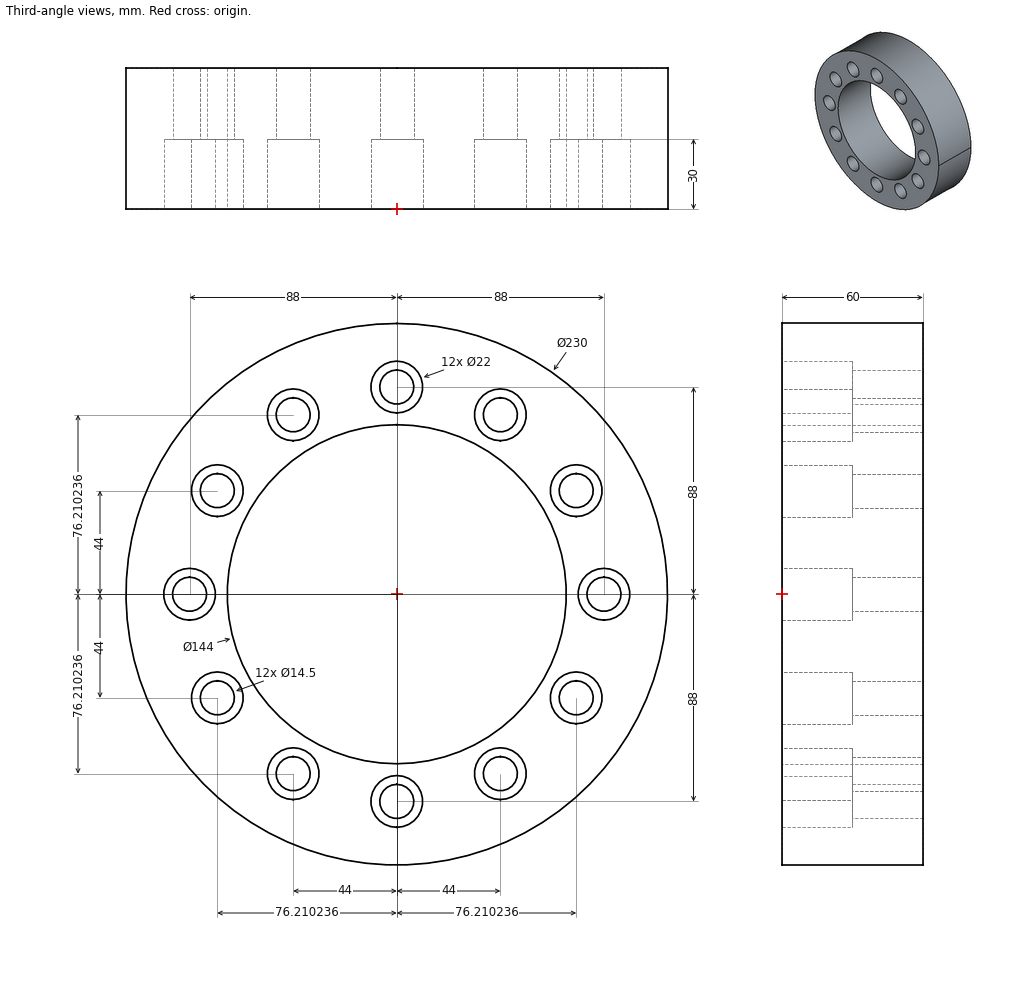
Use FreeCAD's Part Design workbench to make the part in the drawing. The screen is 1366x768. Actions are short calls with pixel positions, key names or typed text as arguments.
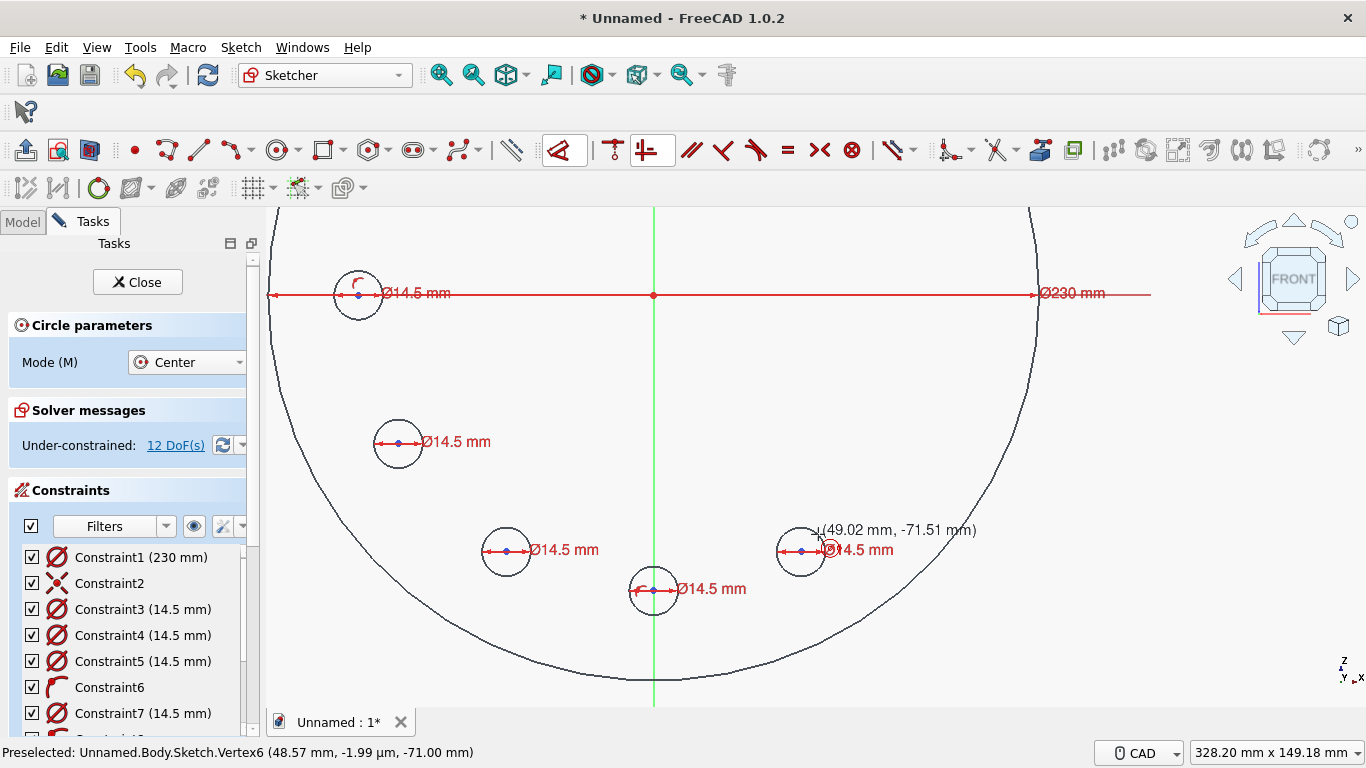
click(909, 443)
move(926, 426)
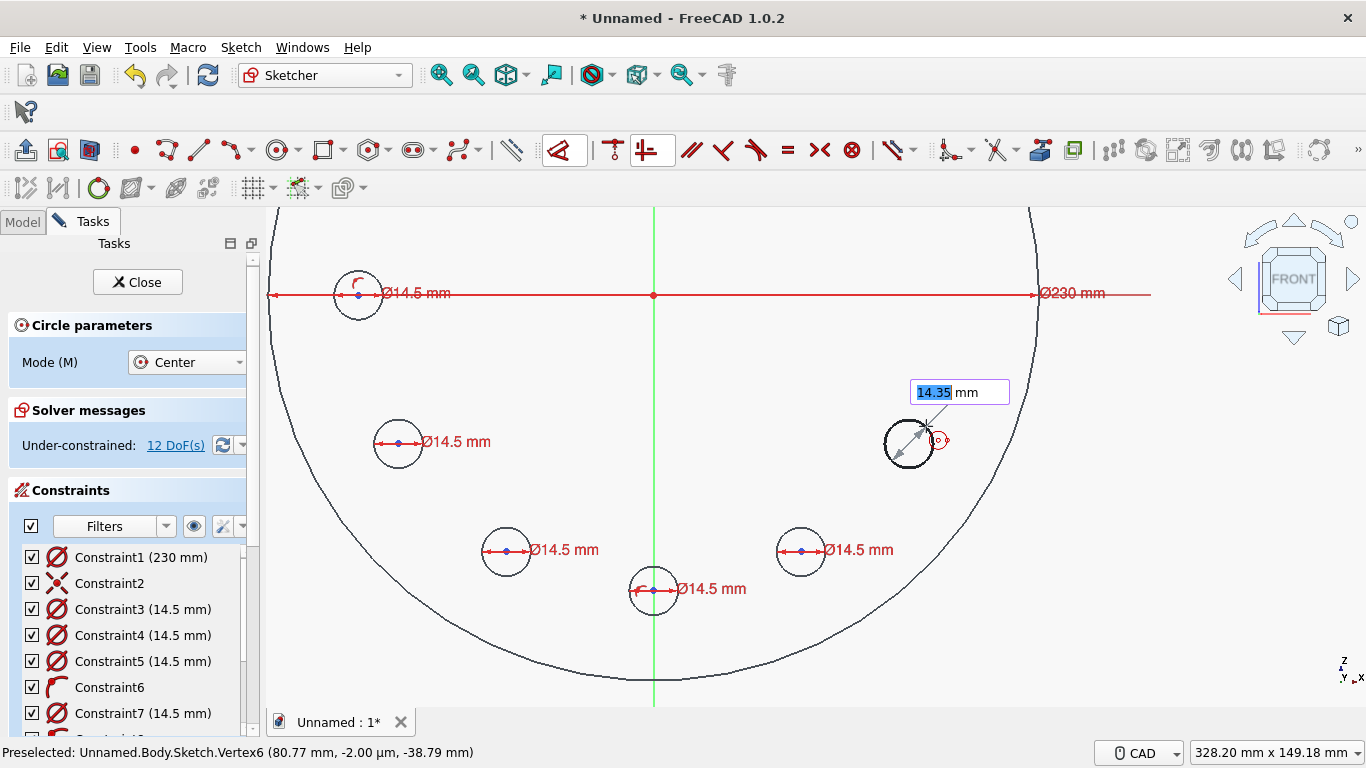
text(14.5)
key(Return)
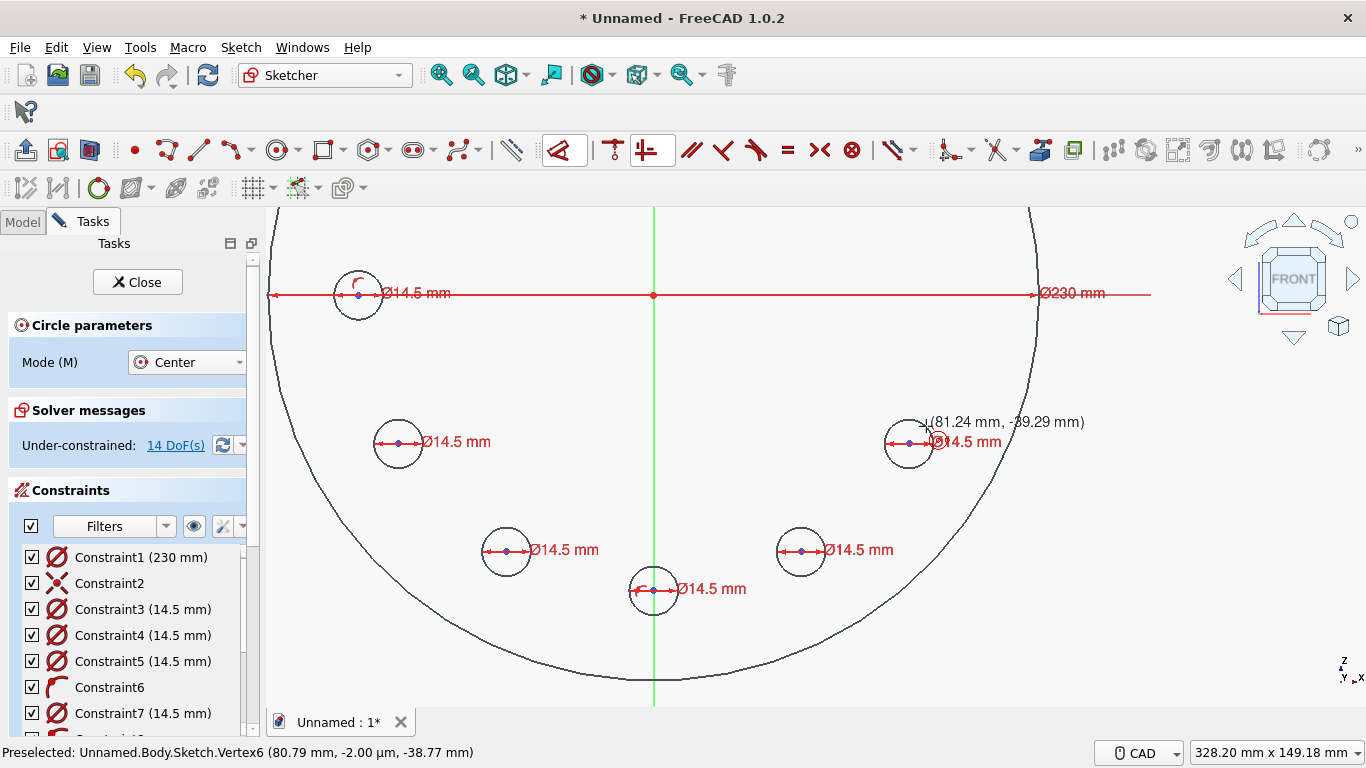
click(949, 295)
move(966, 278)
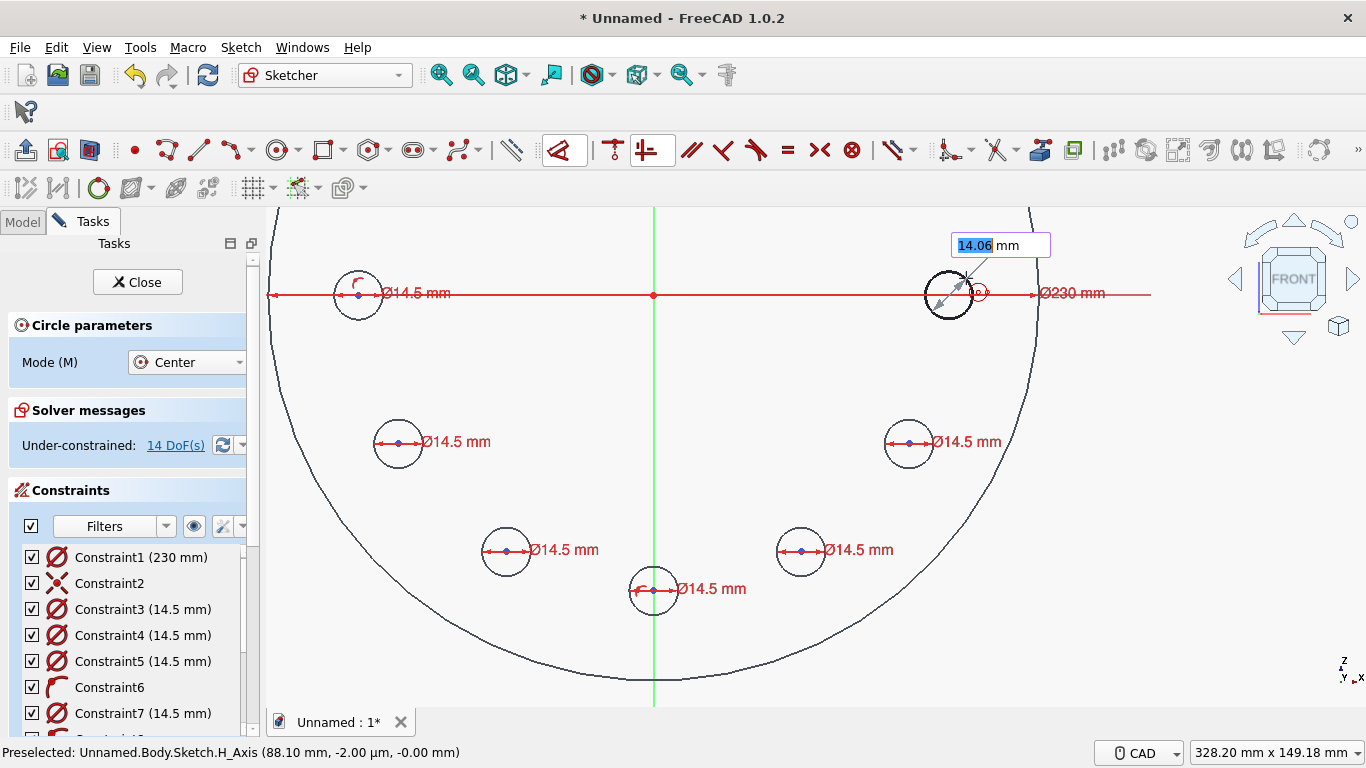
text(14.5)
key(Return)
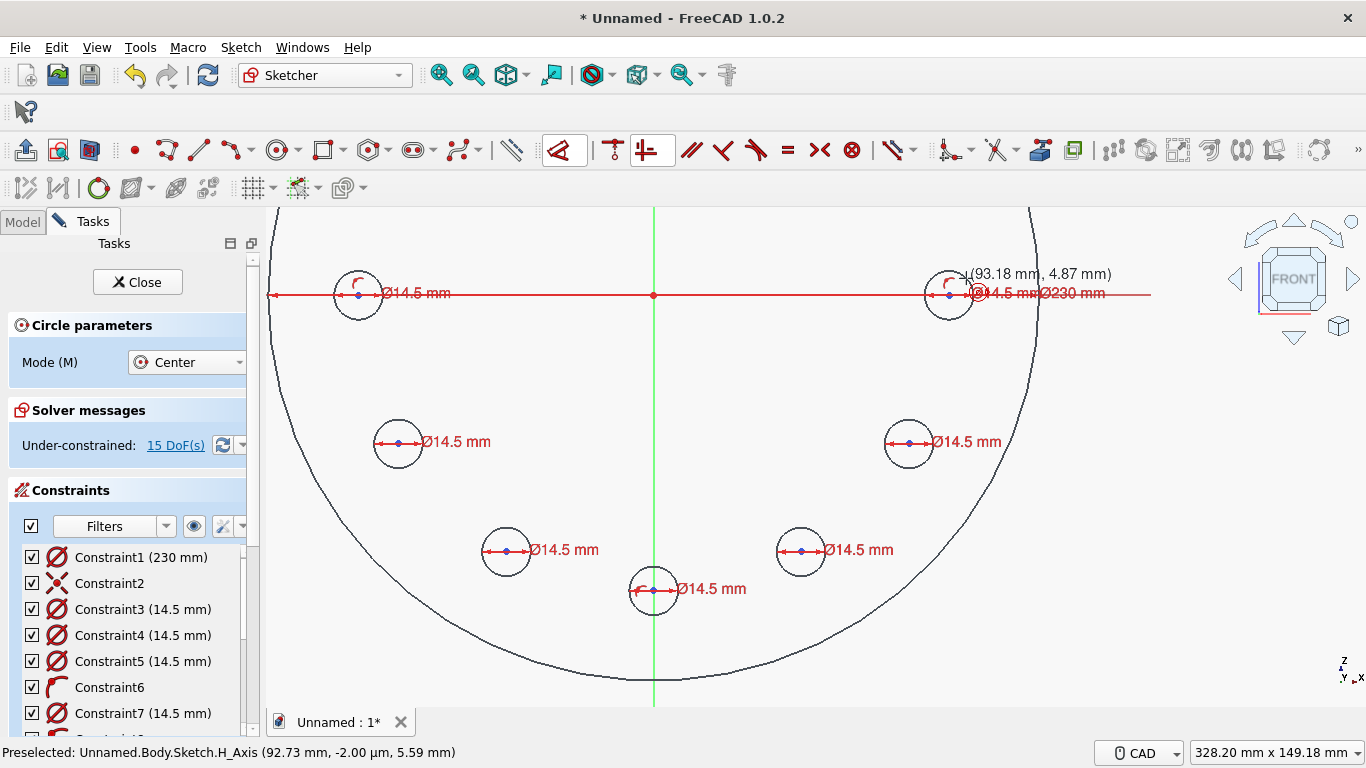
click(654, 295)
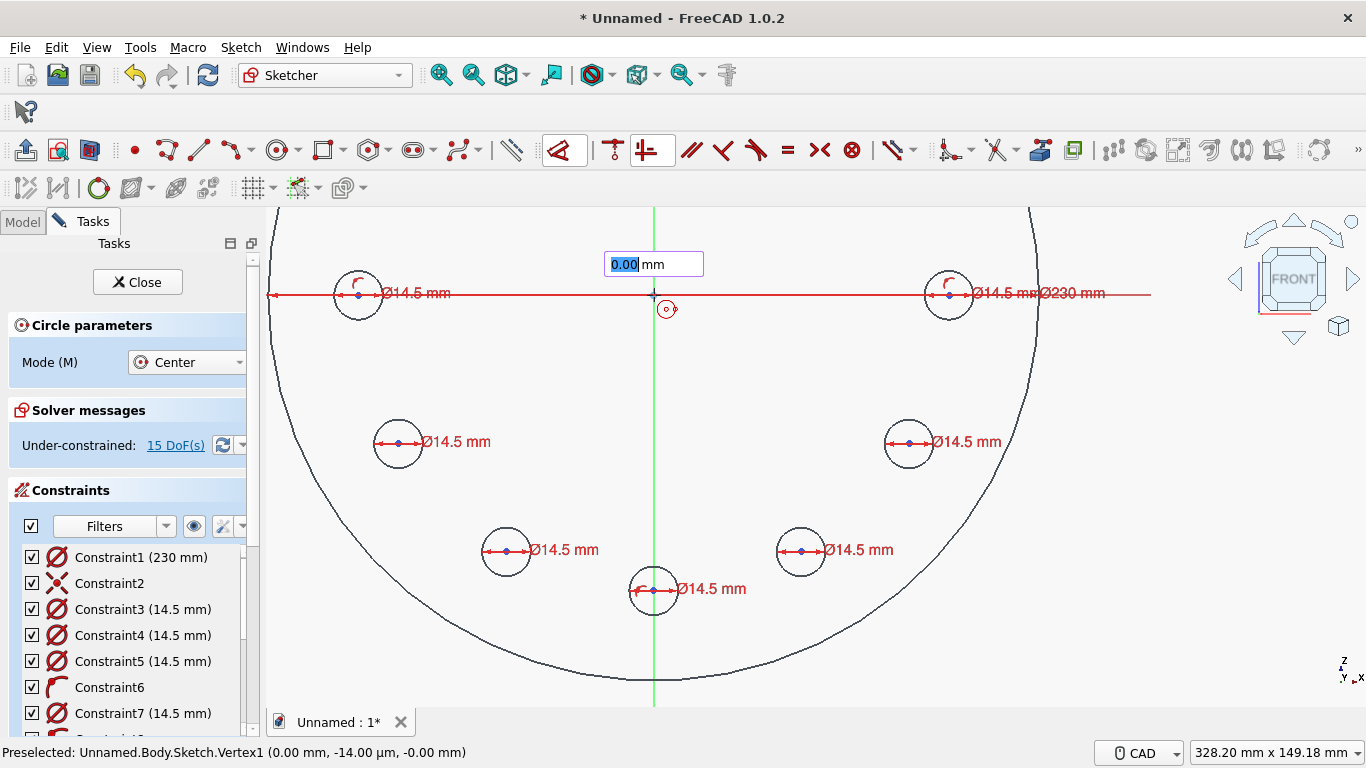
scroll(802, 551, down, 5)
move(811, 395)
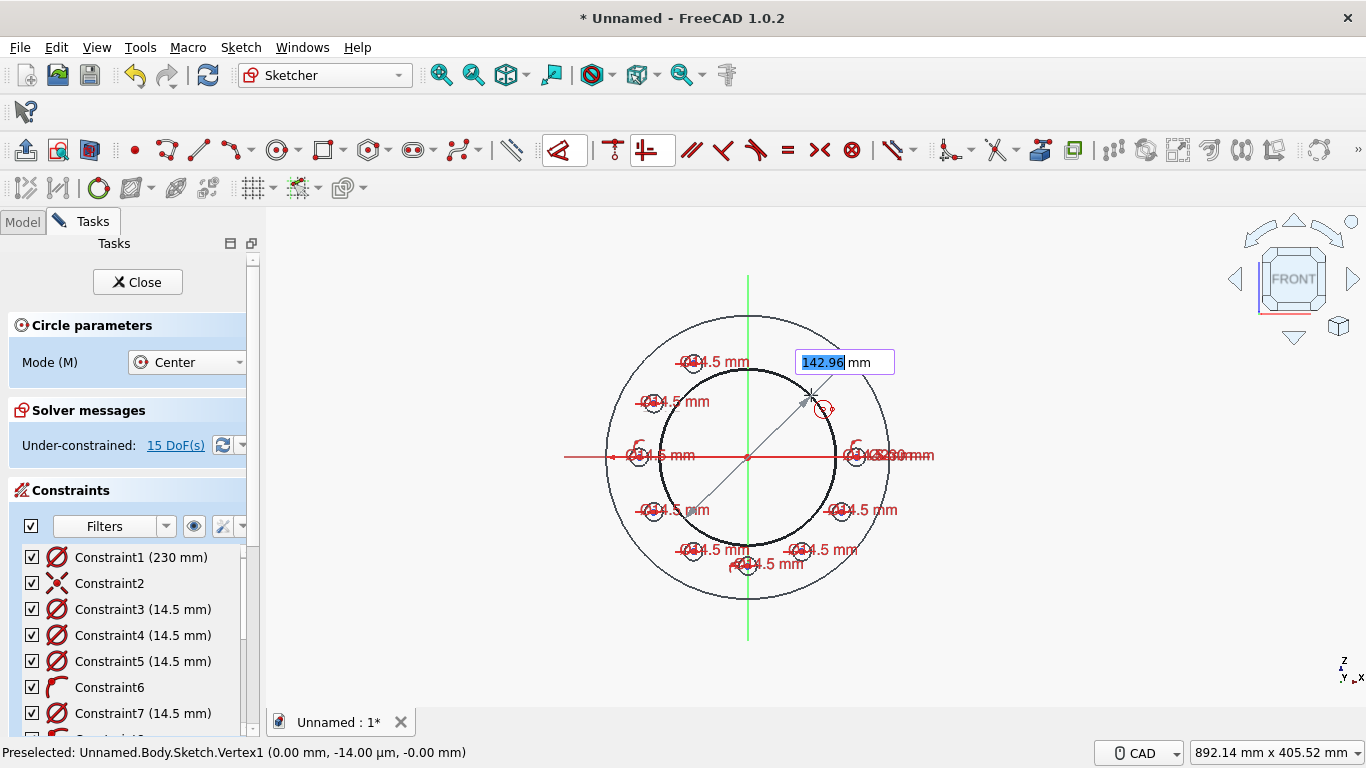
text(144)
key(Return)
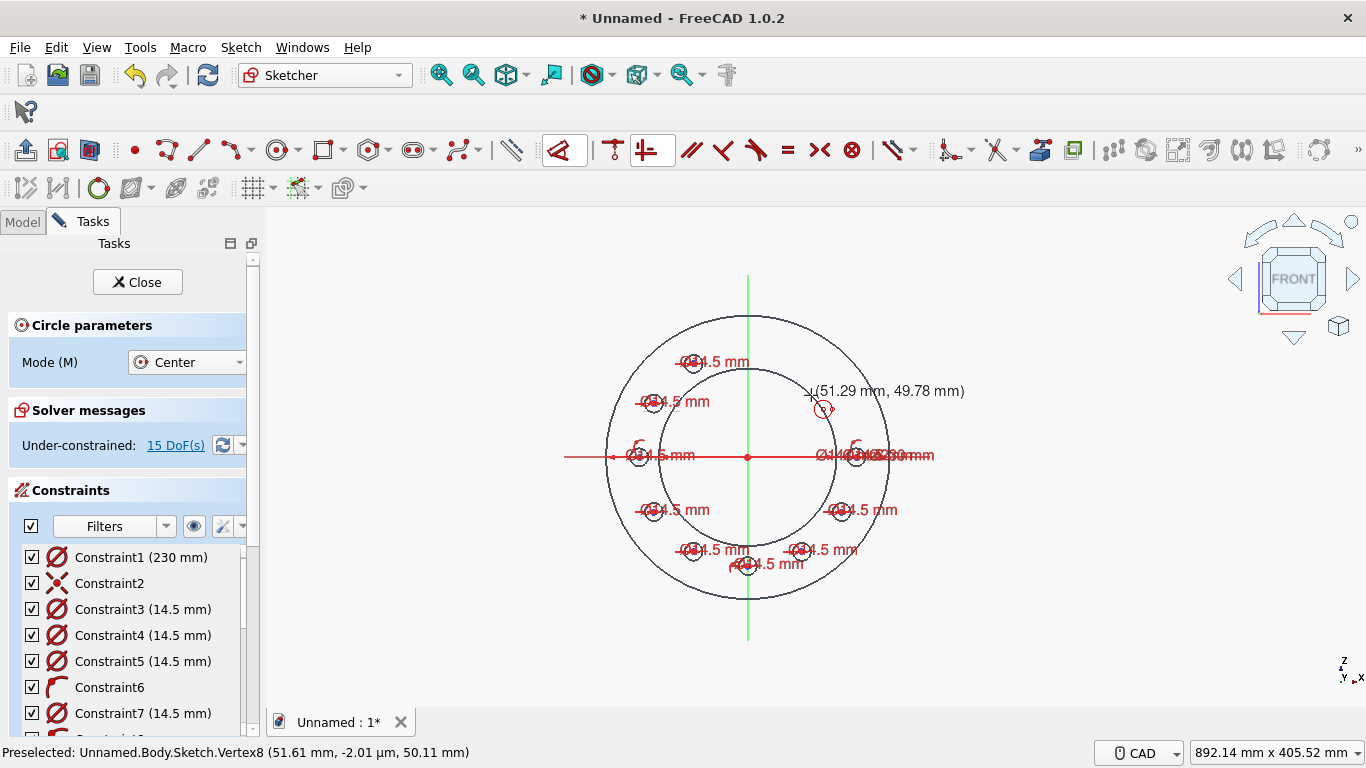
scroll(748, 349, up, 5)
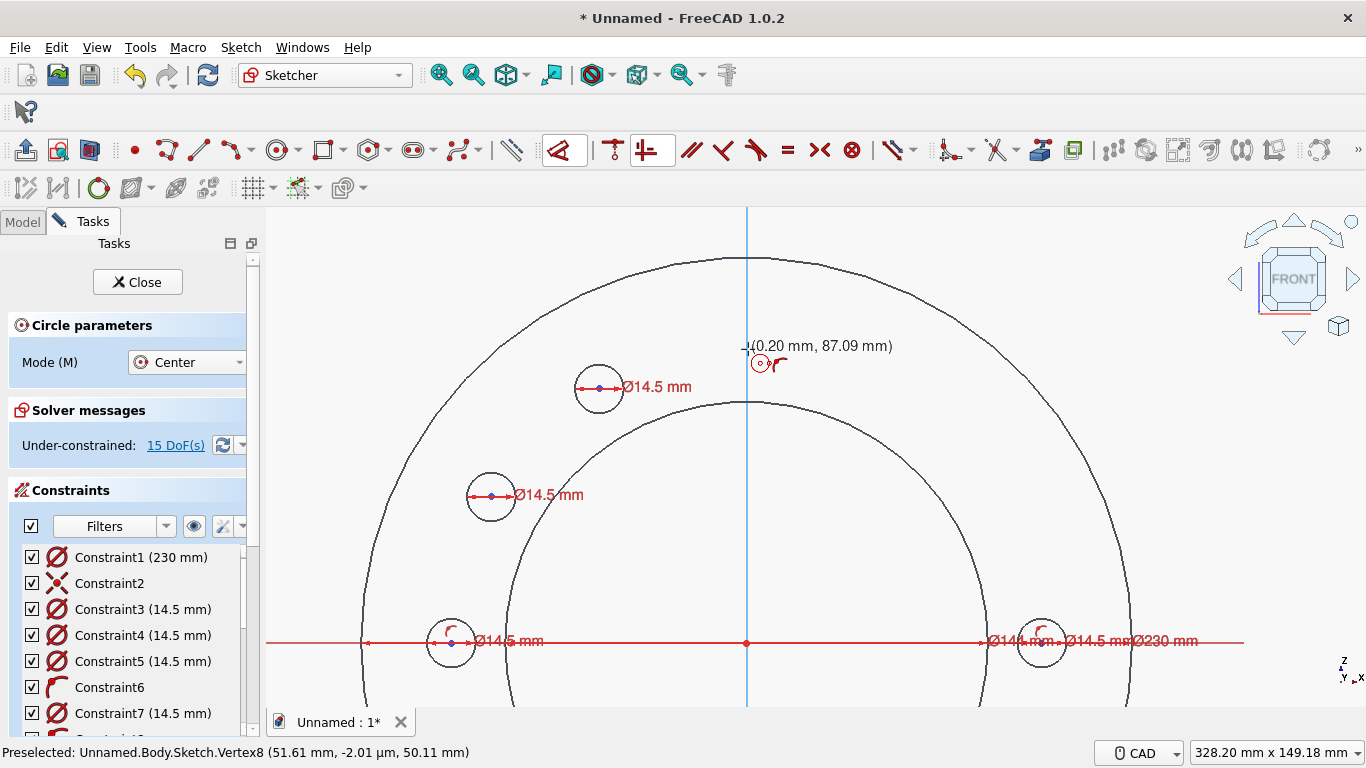
click(747, 348)
move(764, 331)